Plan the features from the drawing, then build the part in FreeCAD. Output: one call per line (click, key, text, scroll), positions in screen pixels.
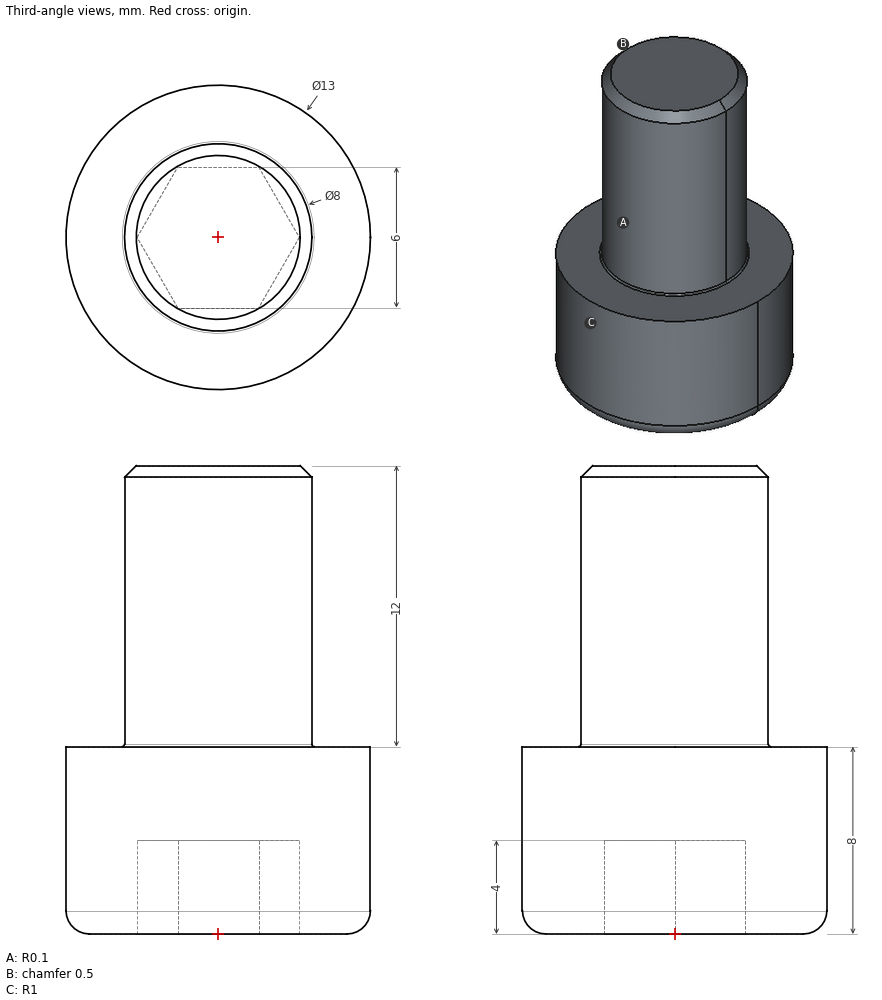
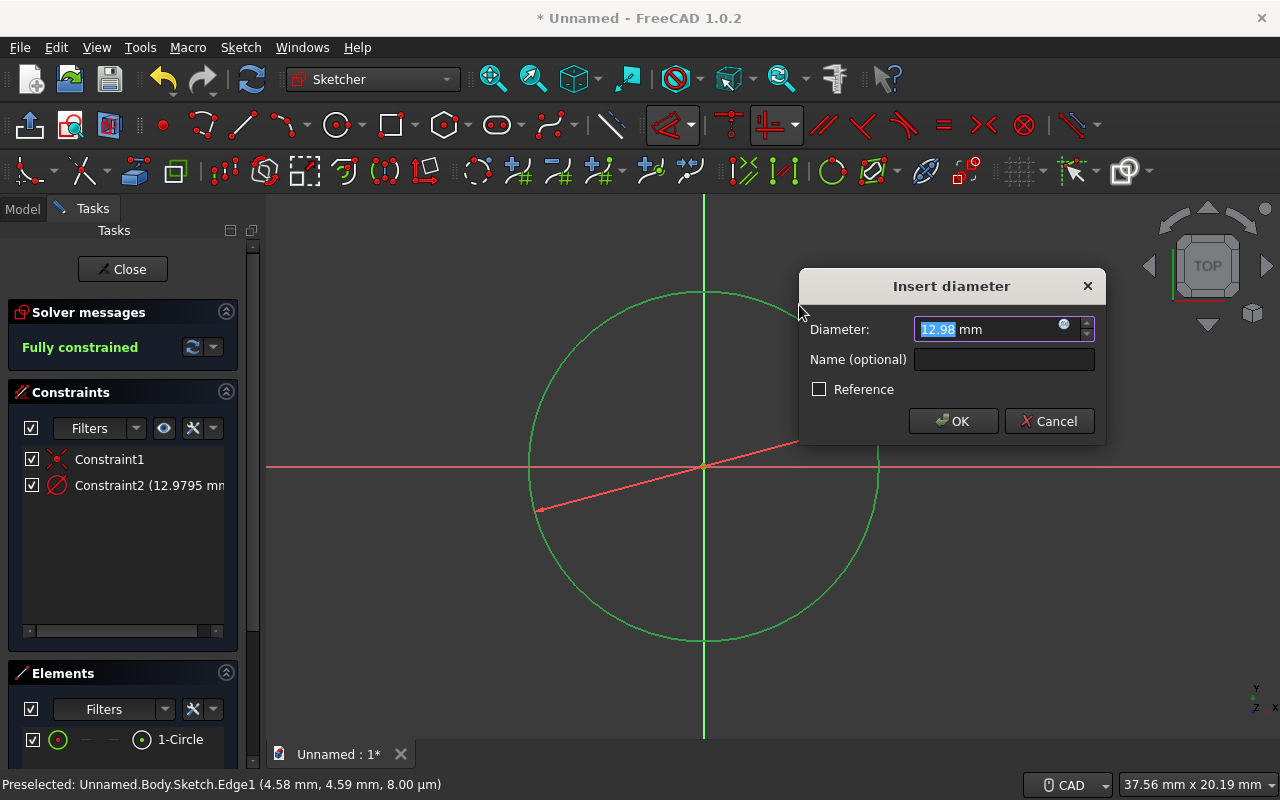
text(13)
key(Return)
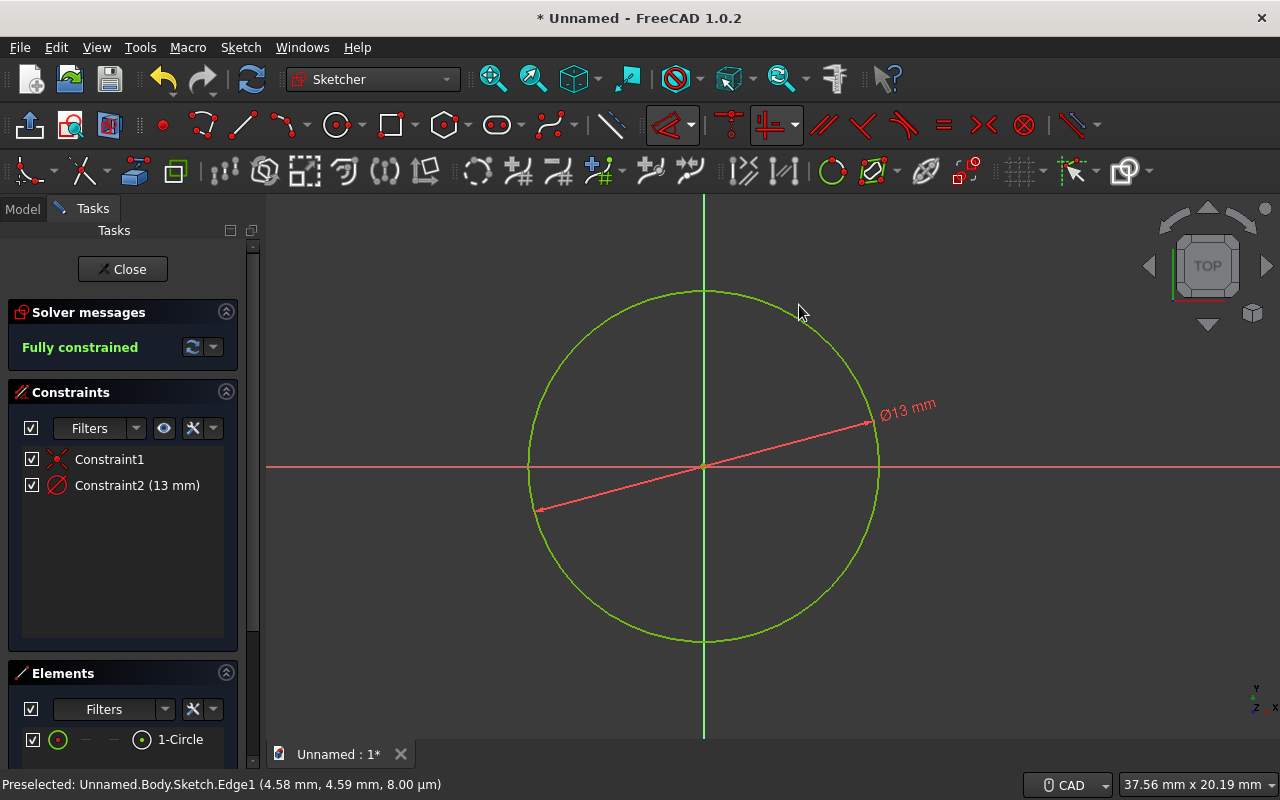
click(123, 269)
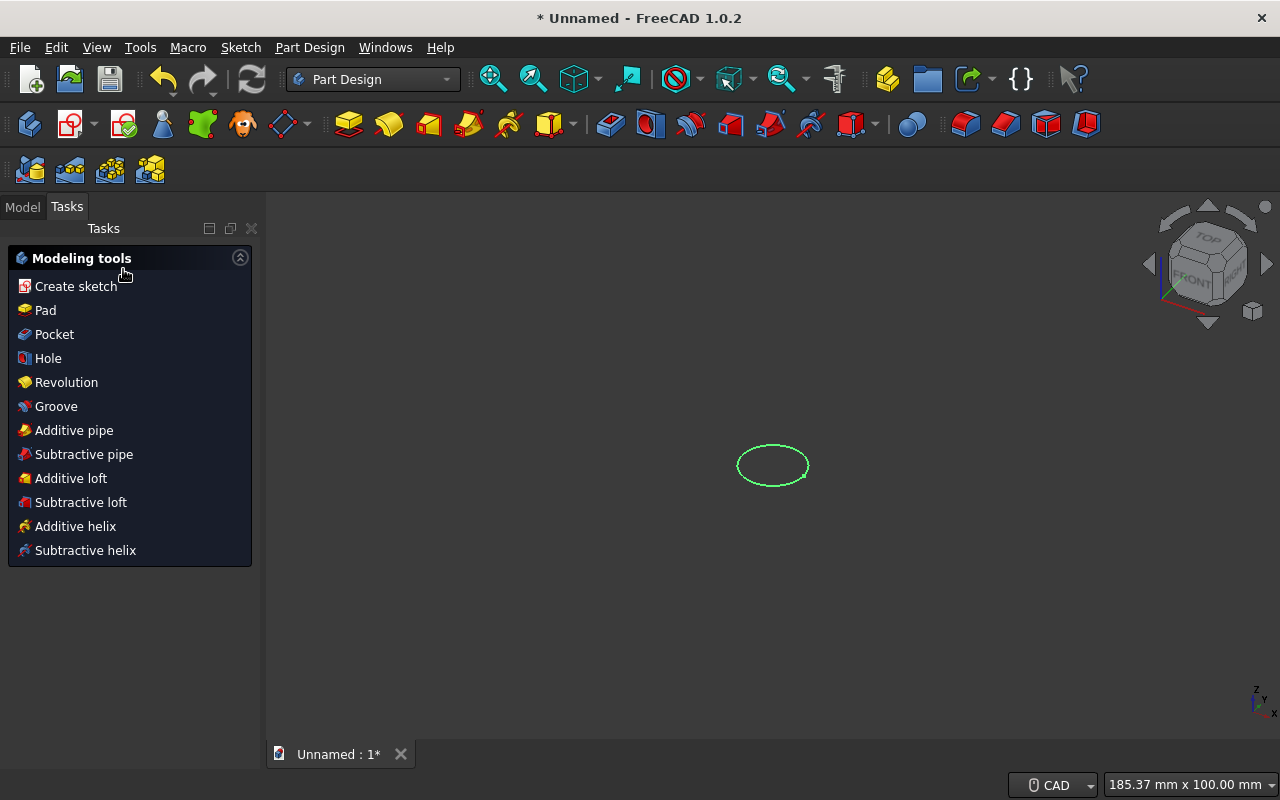
click(350, 124)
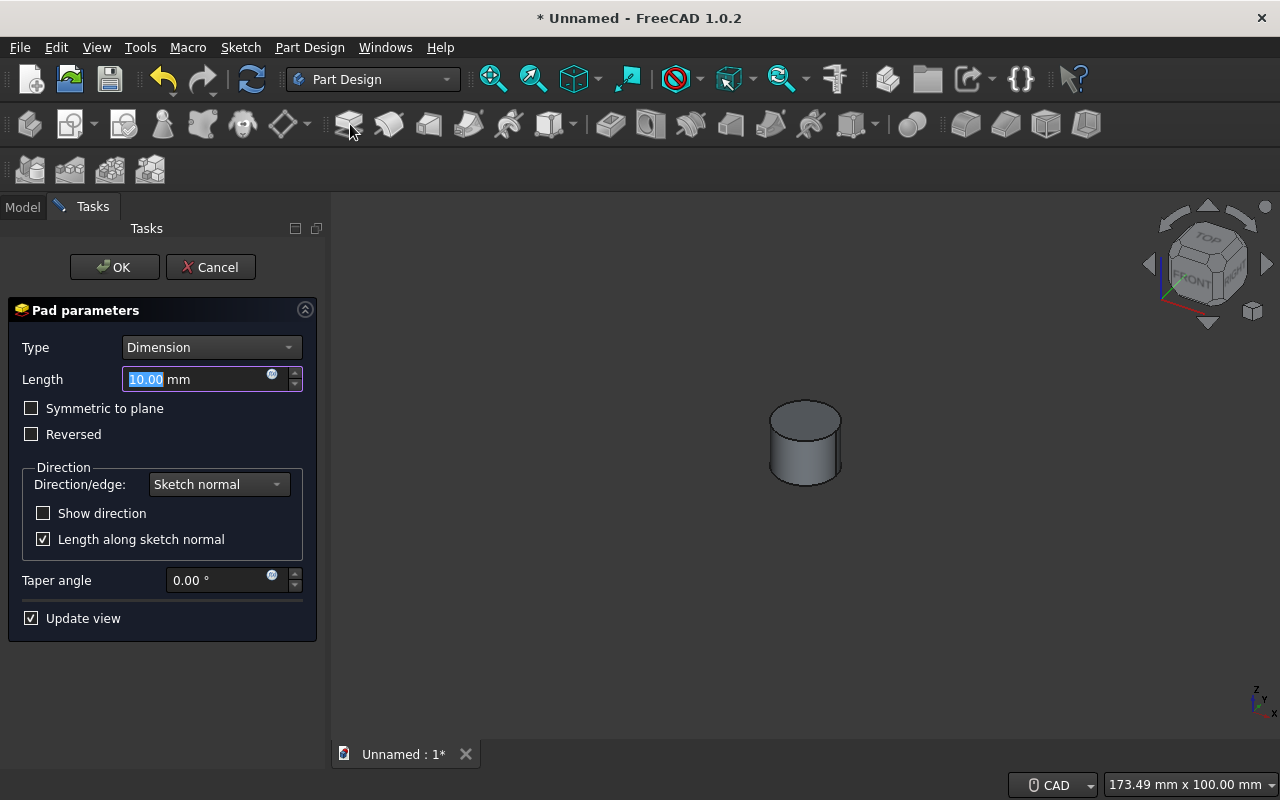
text(8)
key(Tab)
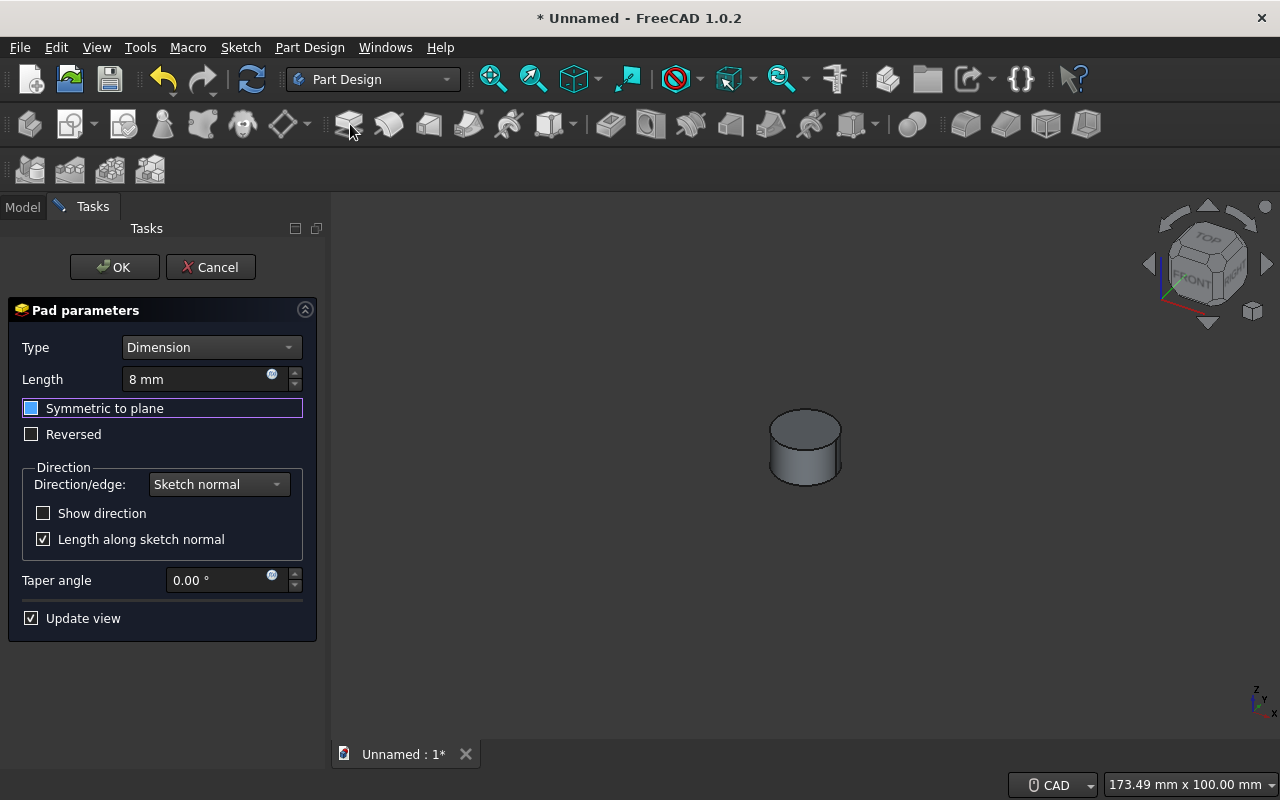
click(115, 267)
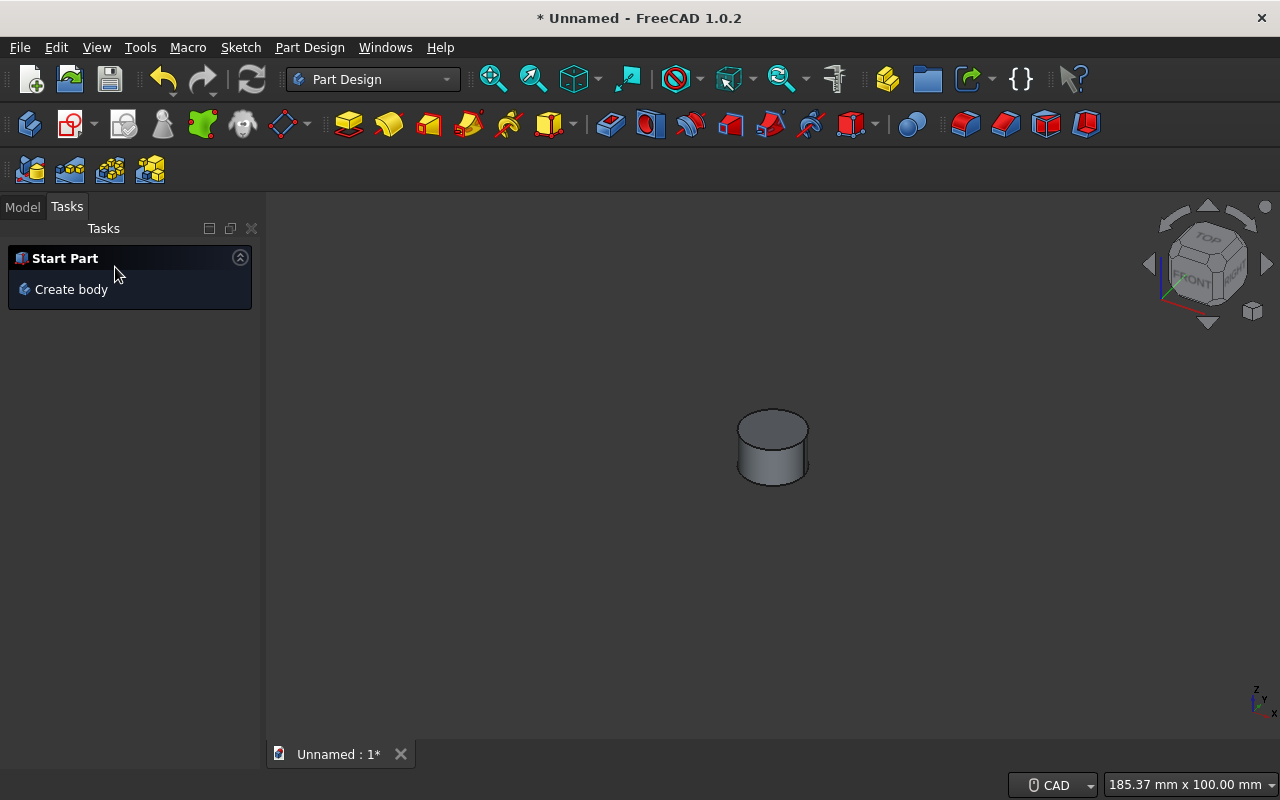
click(494, 80)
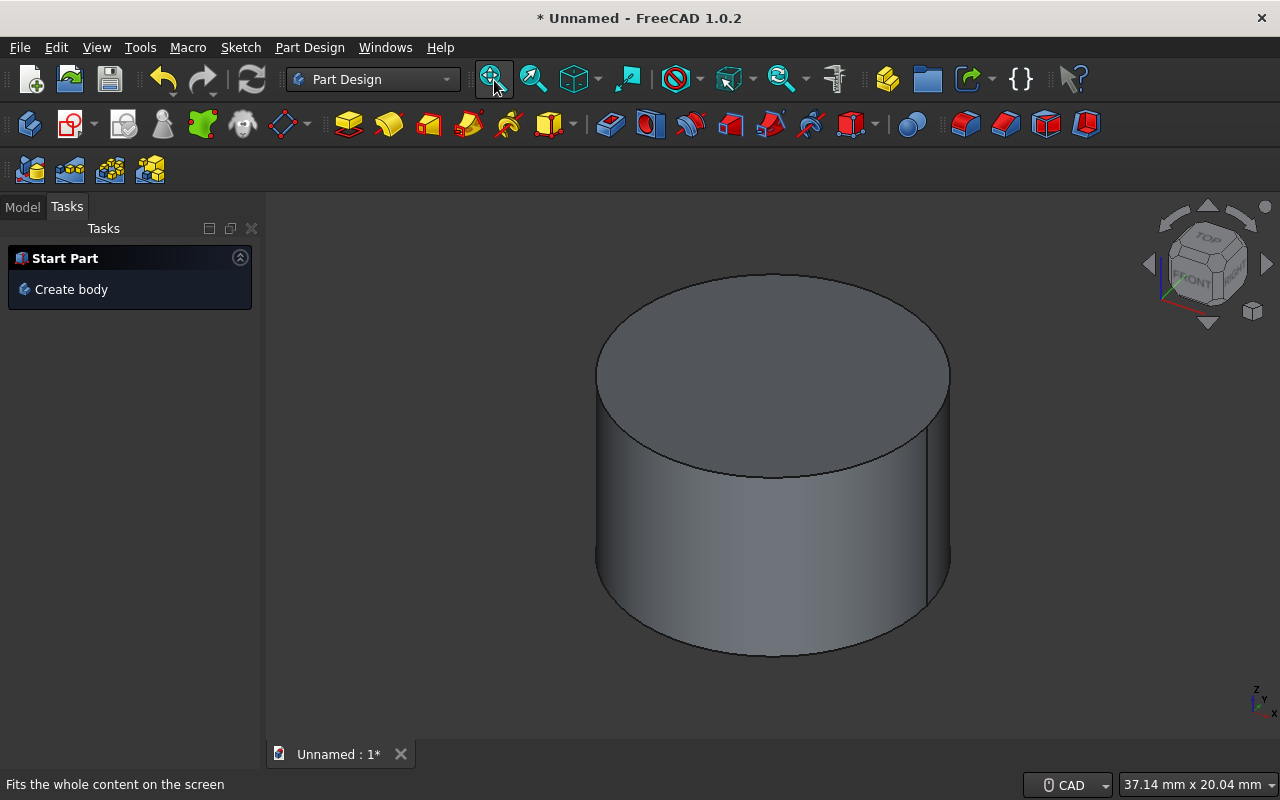
click(773, 375)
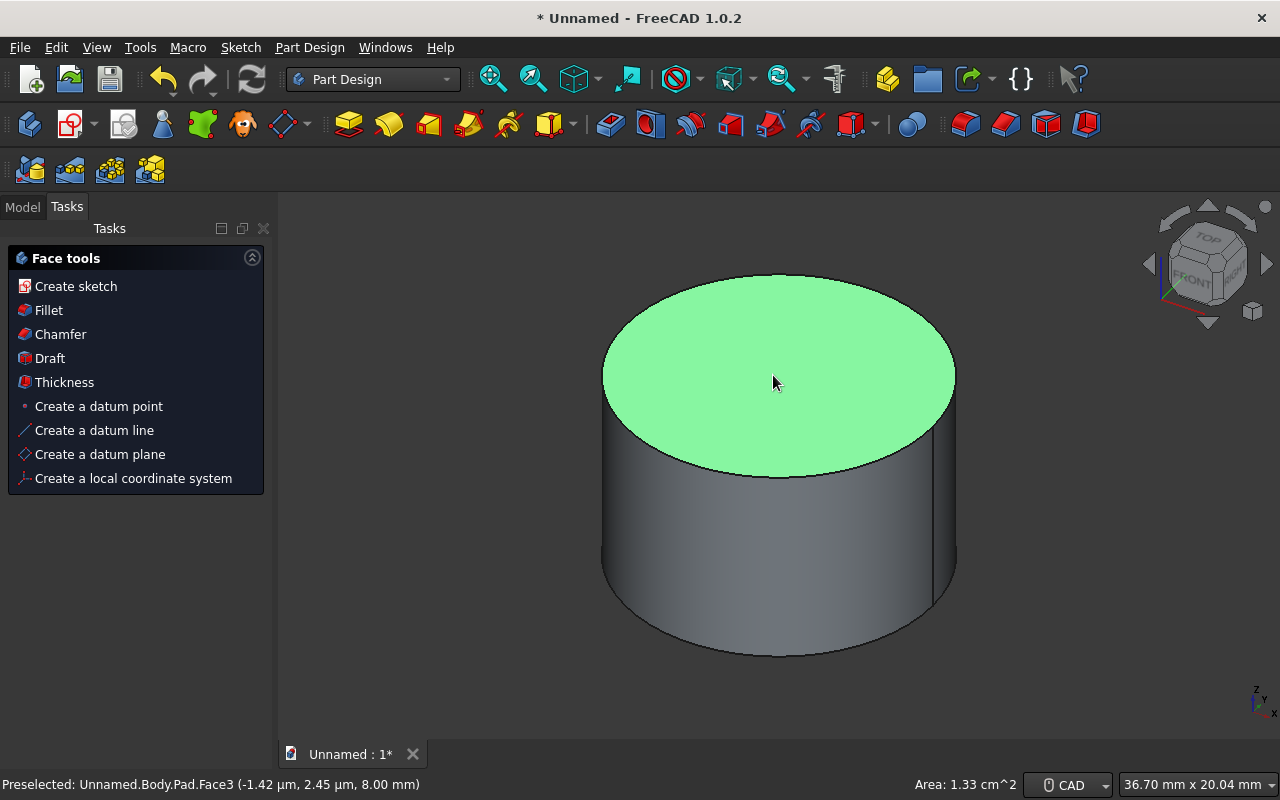
click(70, 124)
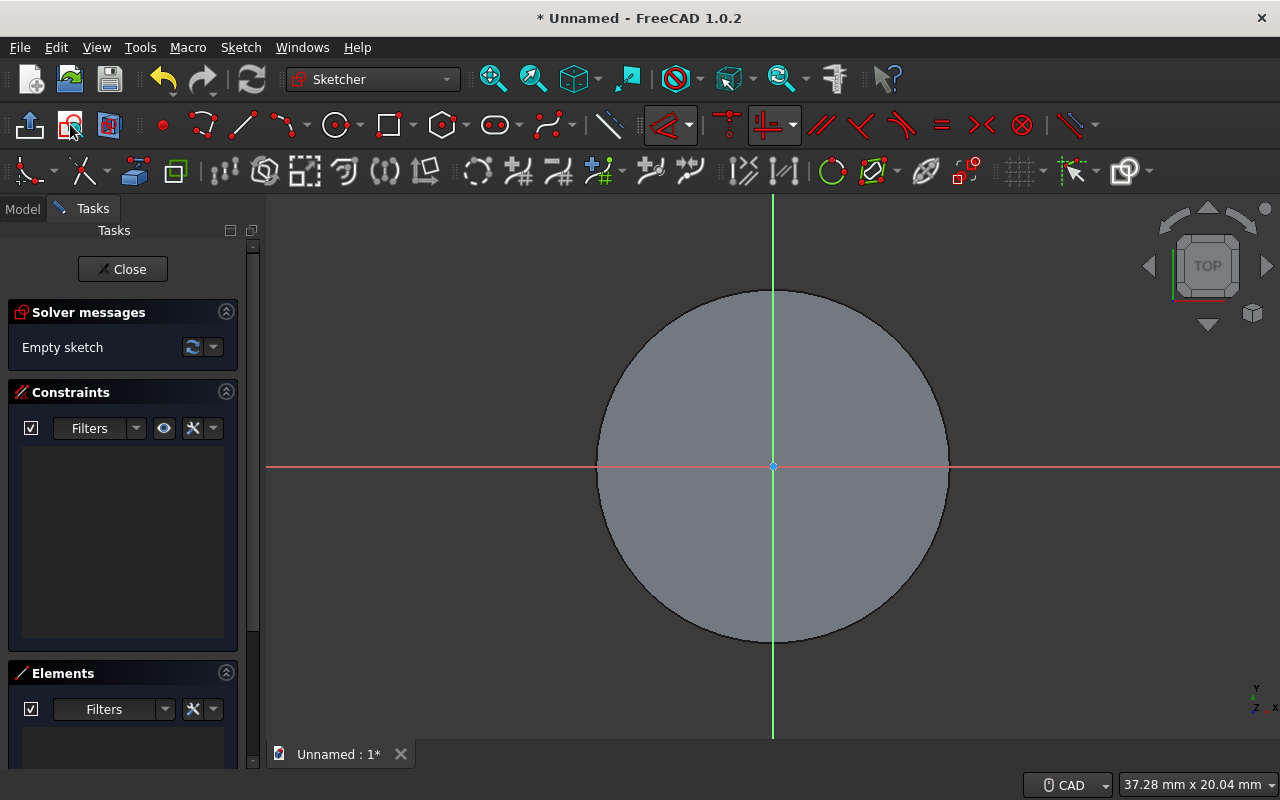
scroll(912, 467, up, 2)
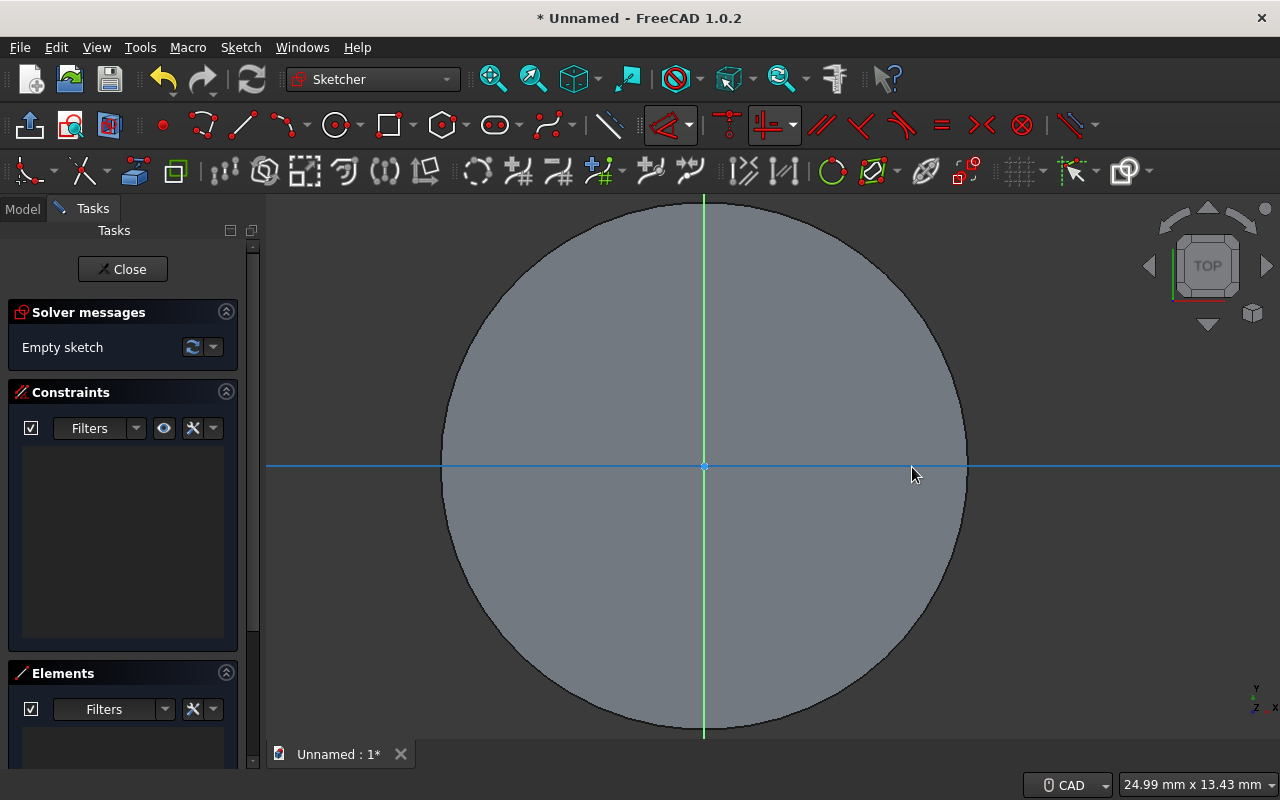
click(336, 126)